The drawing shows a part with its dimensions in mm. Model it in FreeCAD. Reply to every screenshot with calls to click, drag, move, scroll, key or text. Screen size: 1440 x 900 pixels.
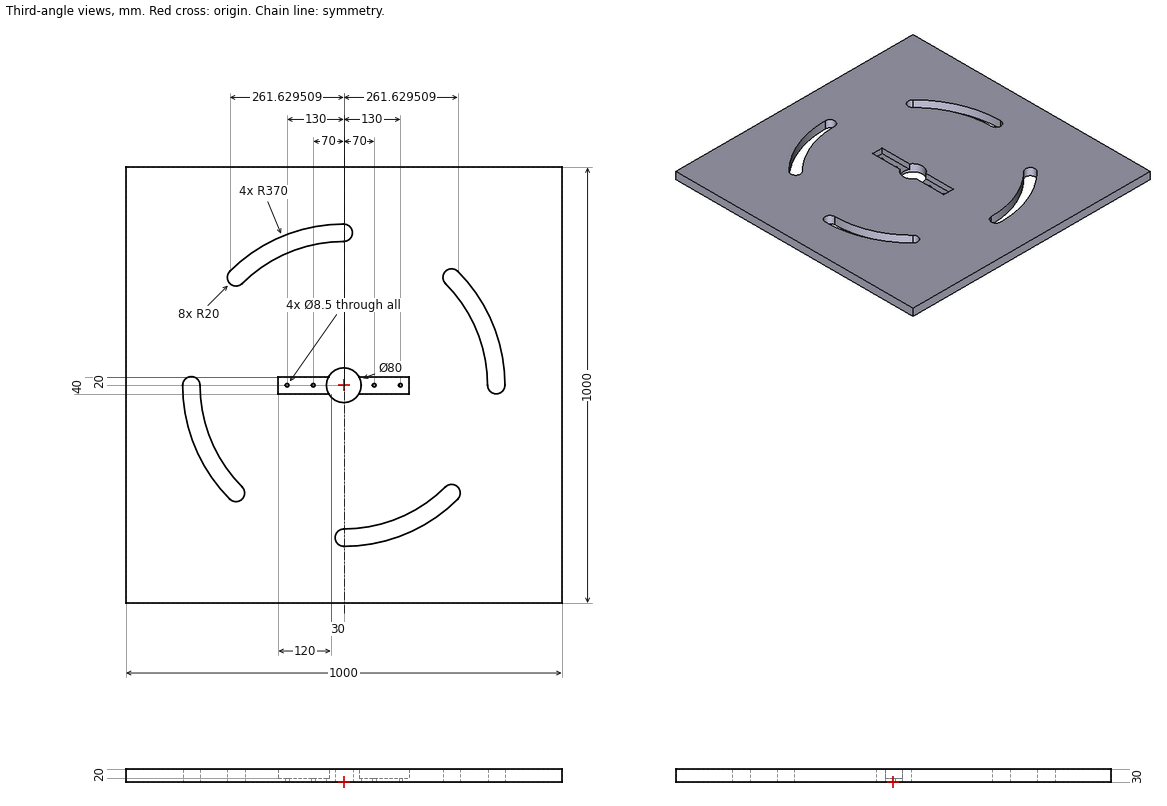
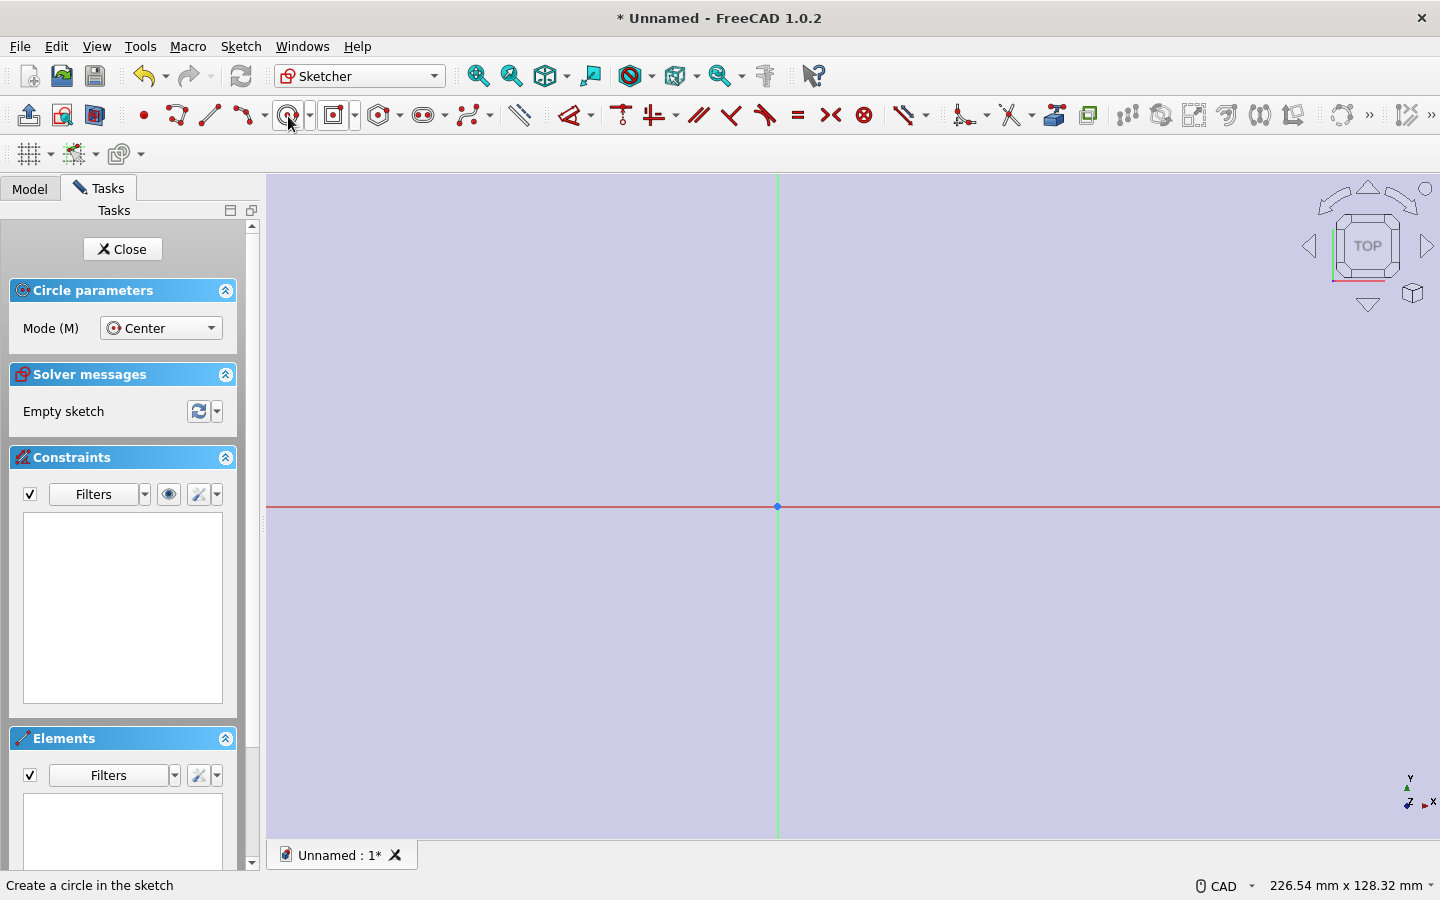
click(778, 506)
click(924, 360)
key(Escape)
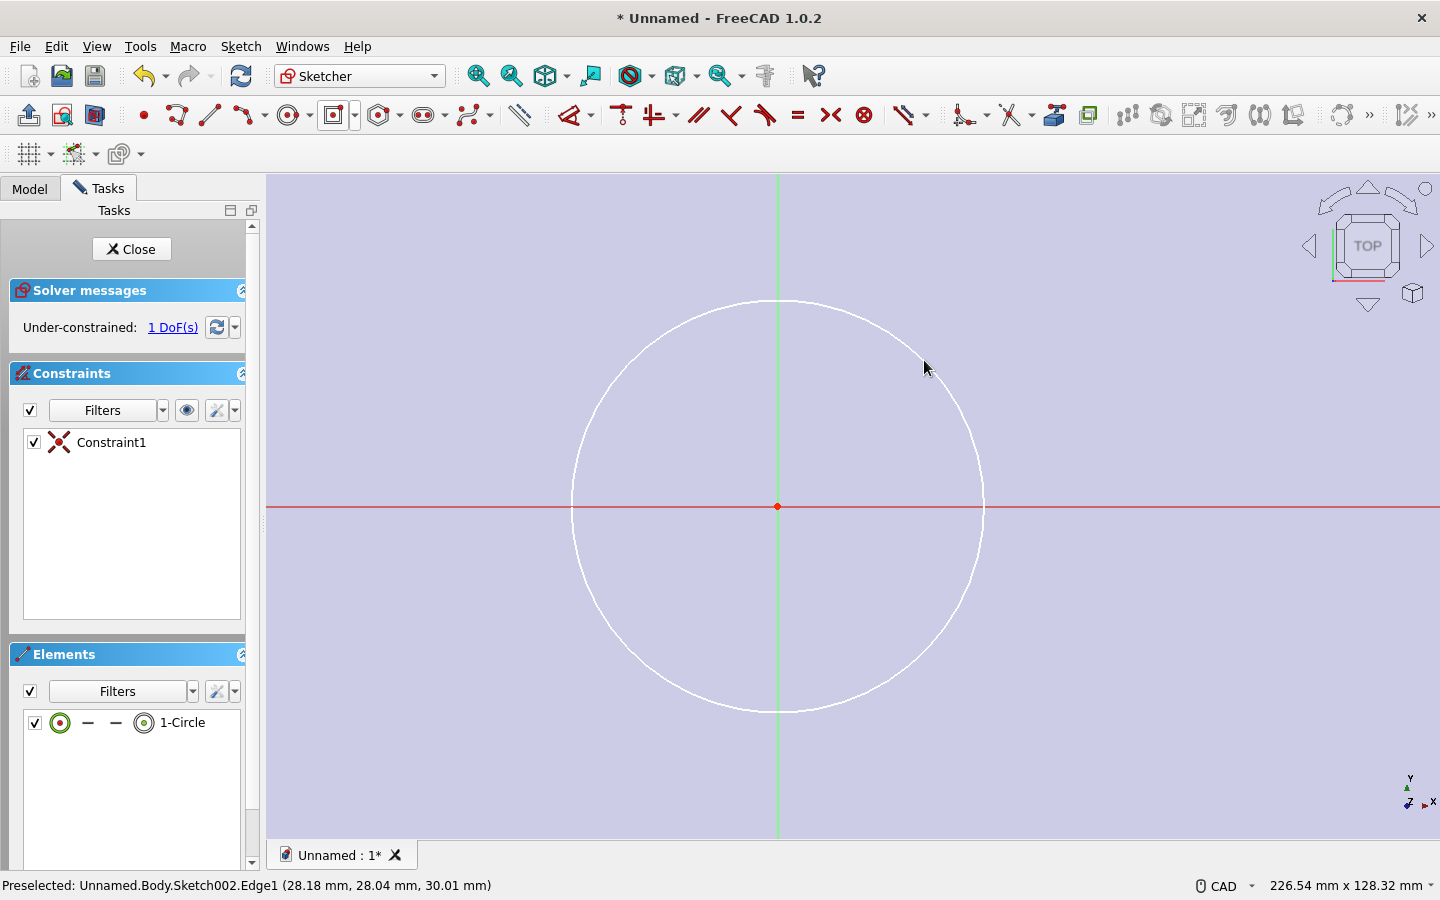
click(568, 116)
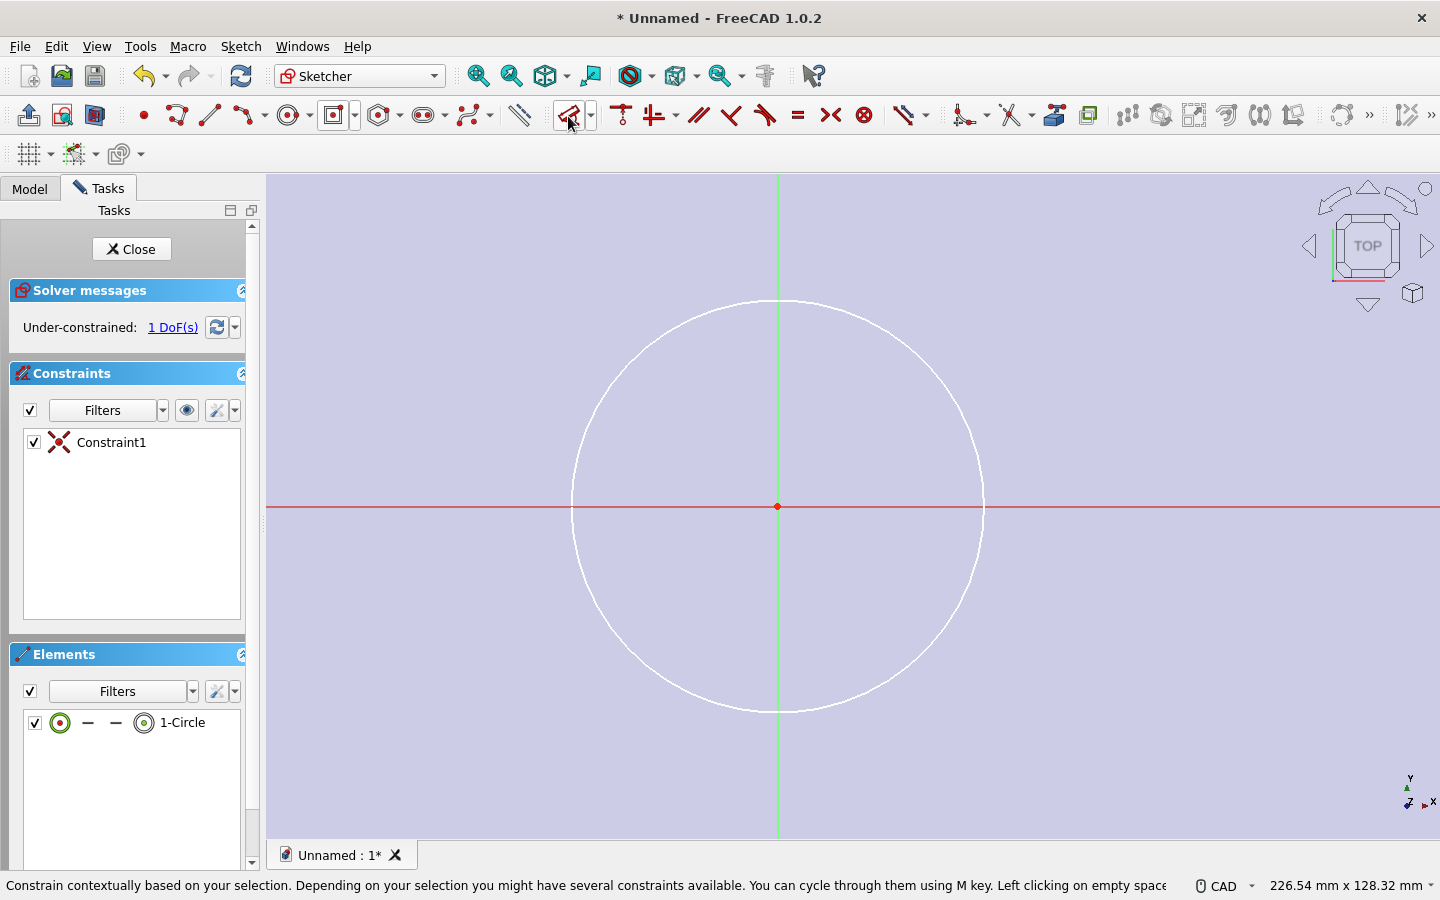
click(923, 360)
click(946, 337)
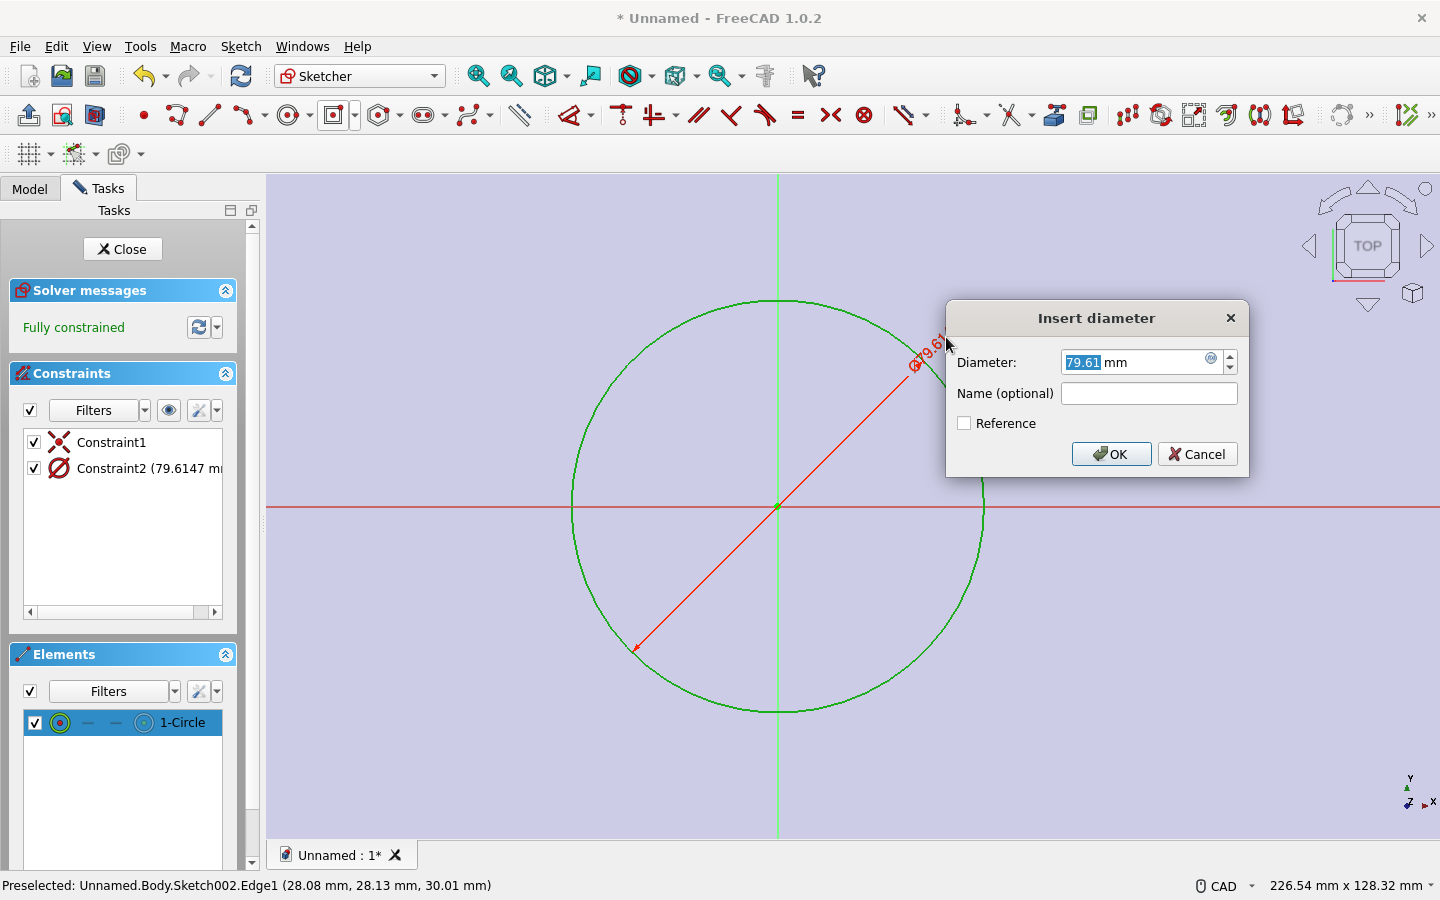
text(80)
key(Return)
key(Escape)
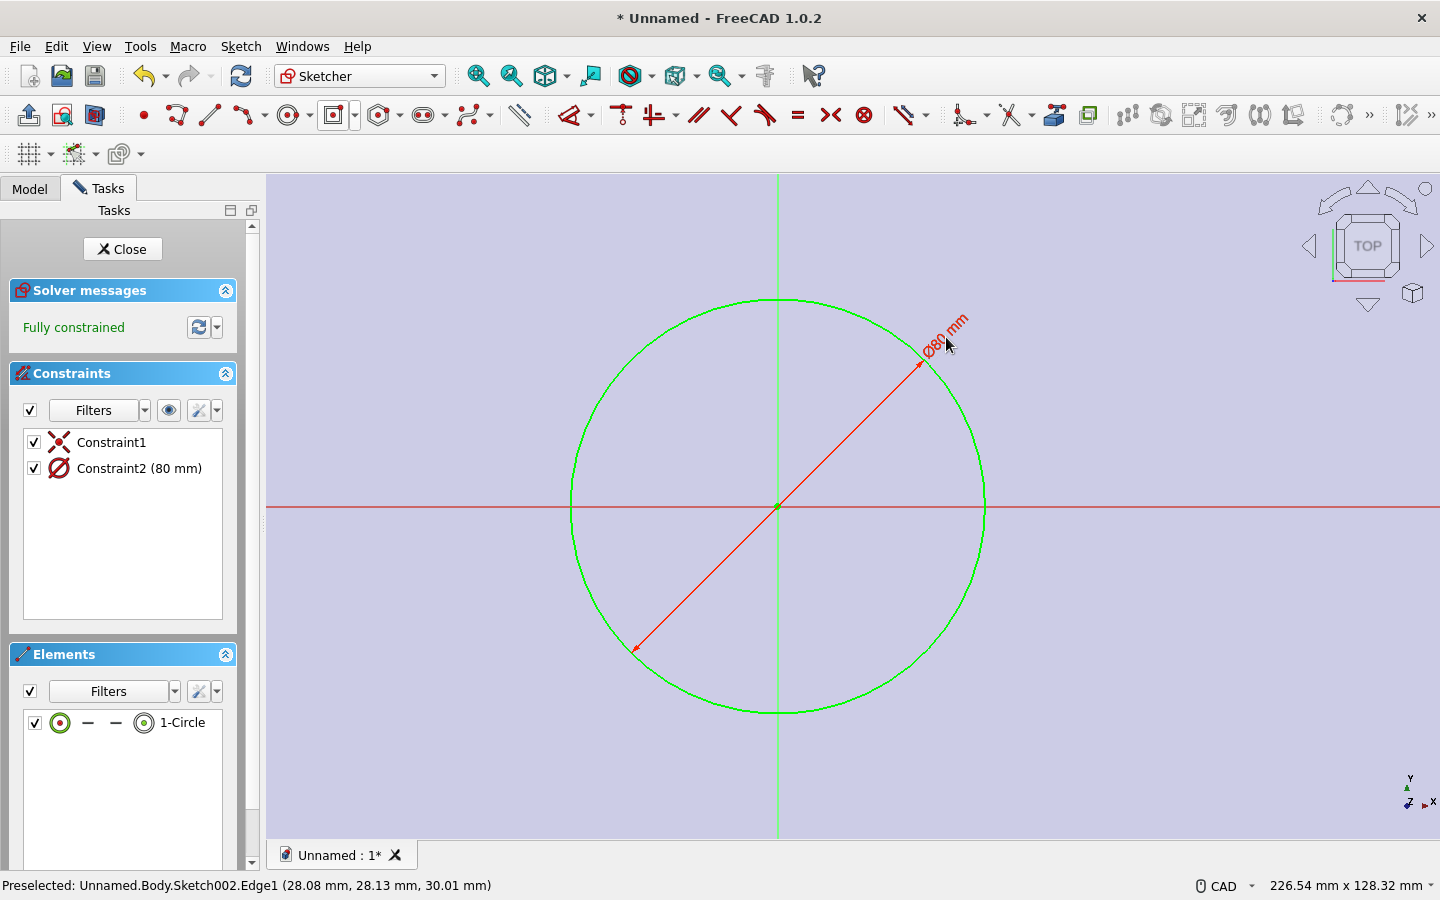
click(123, 249)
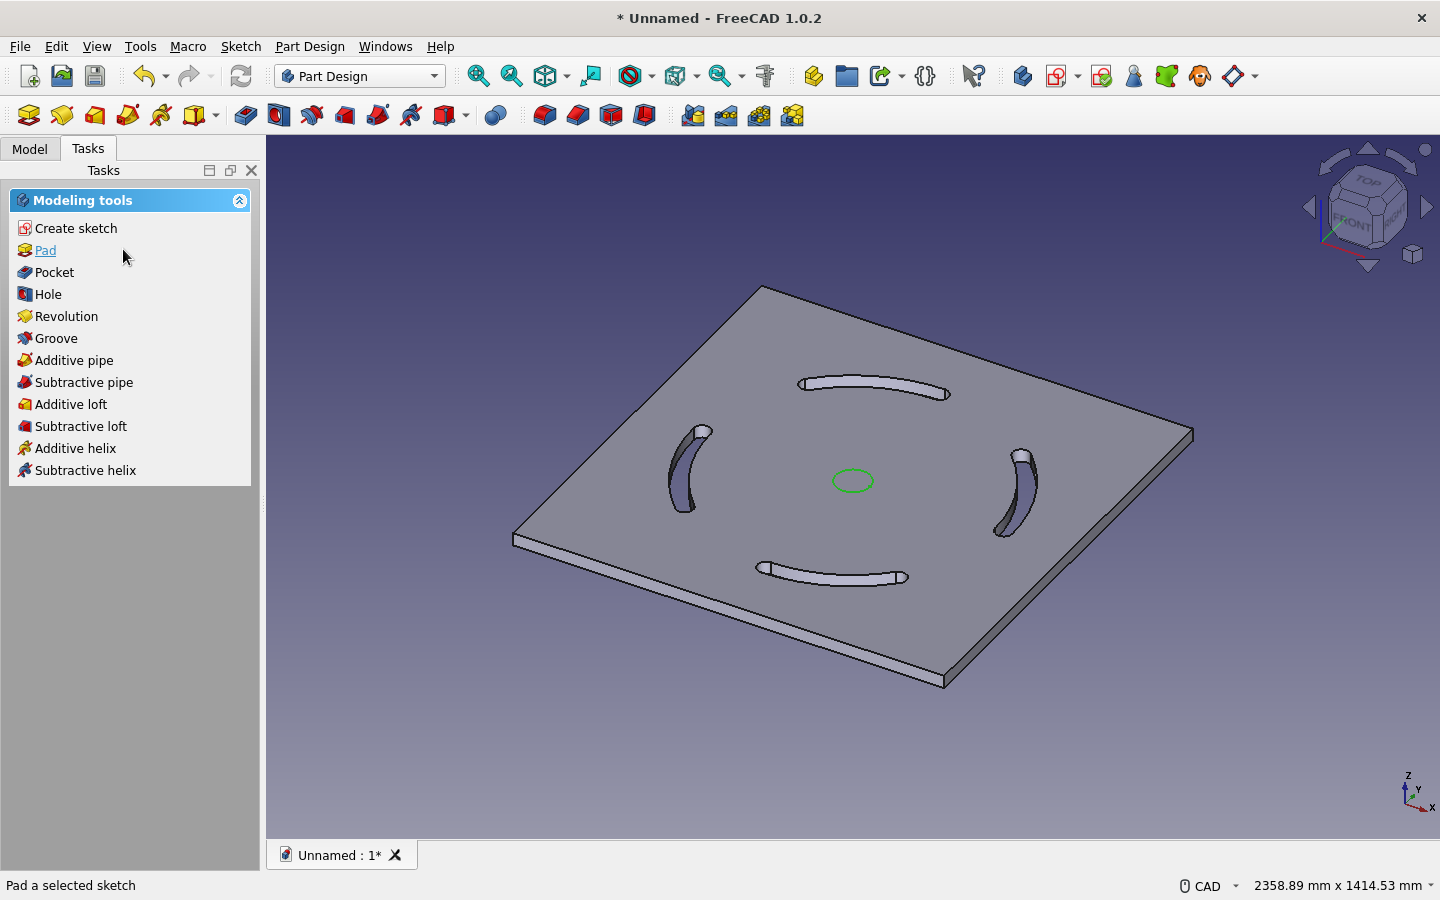
click(246, 116)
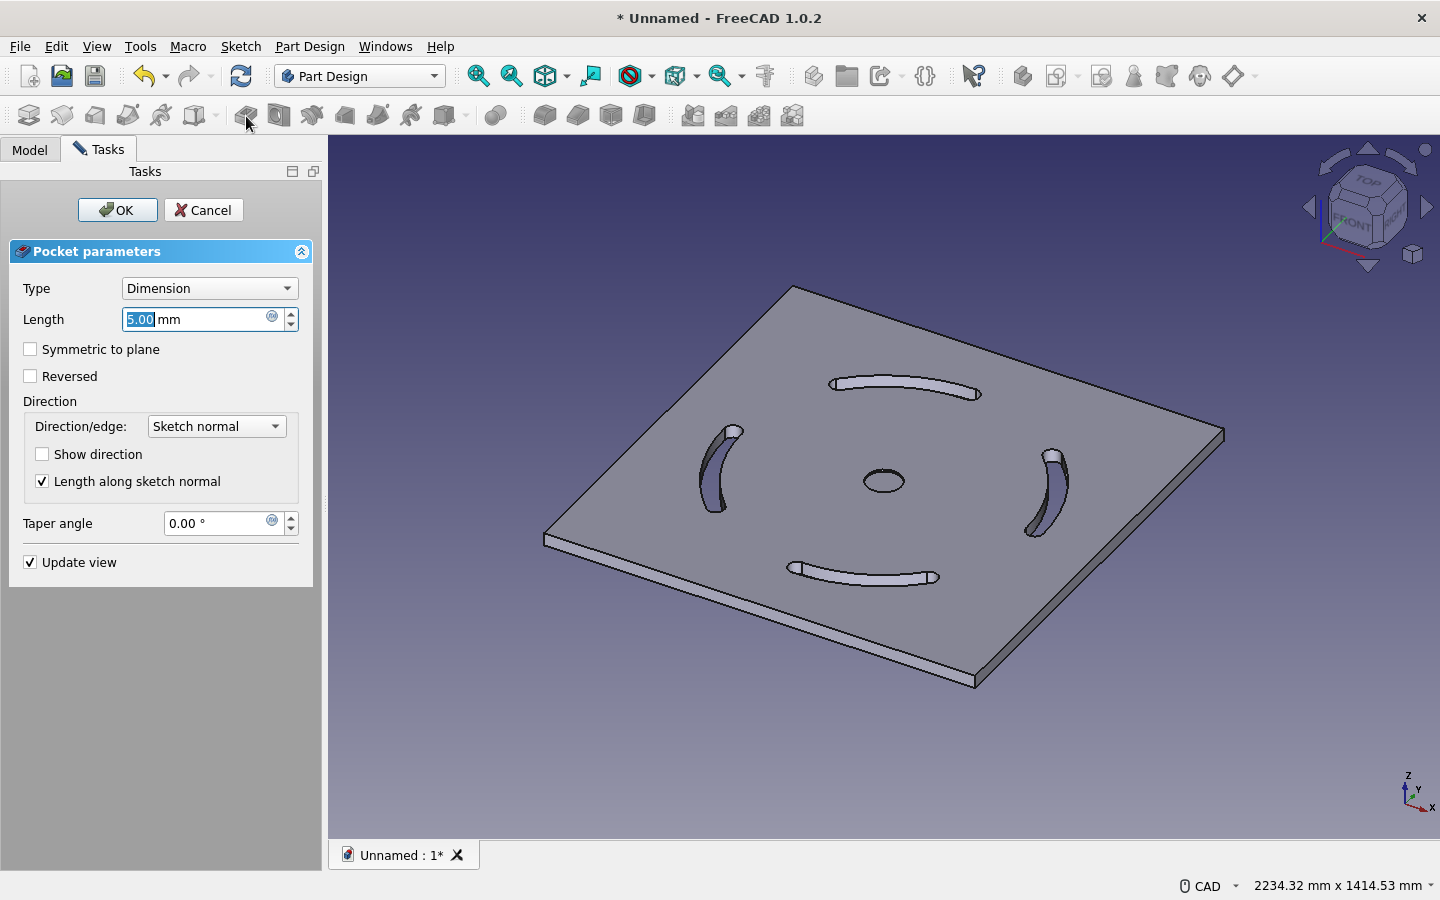
click(210, 288)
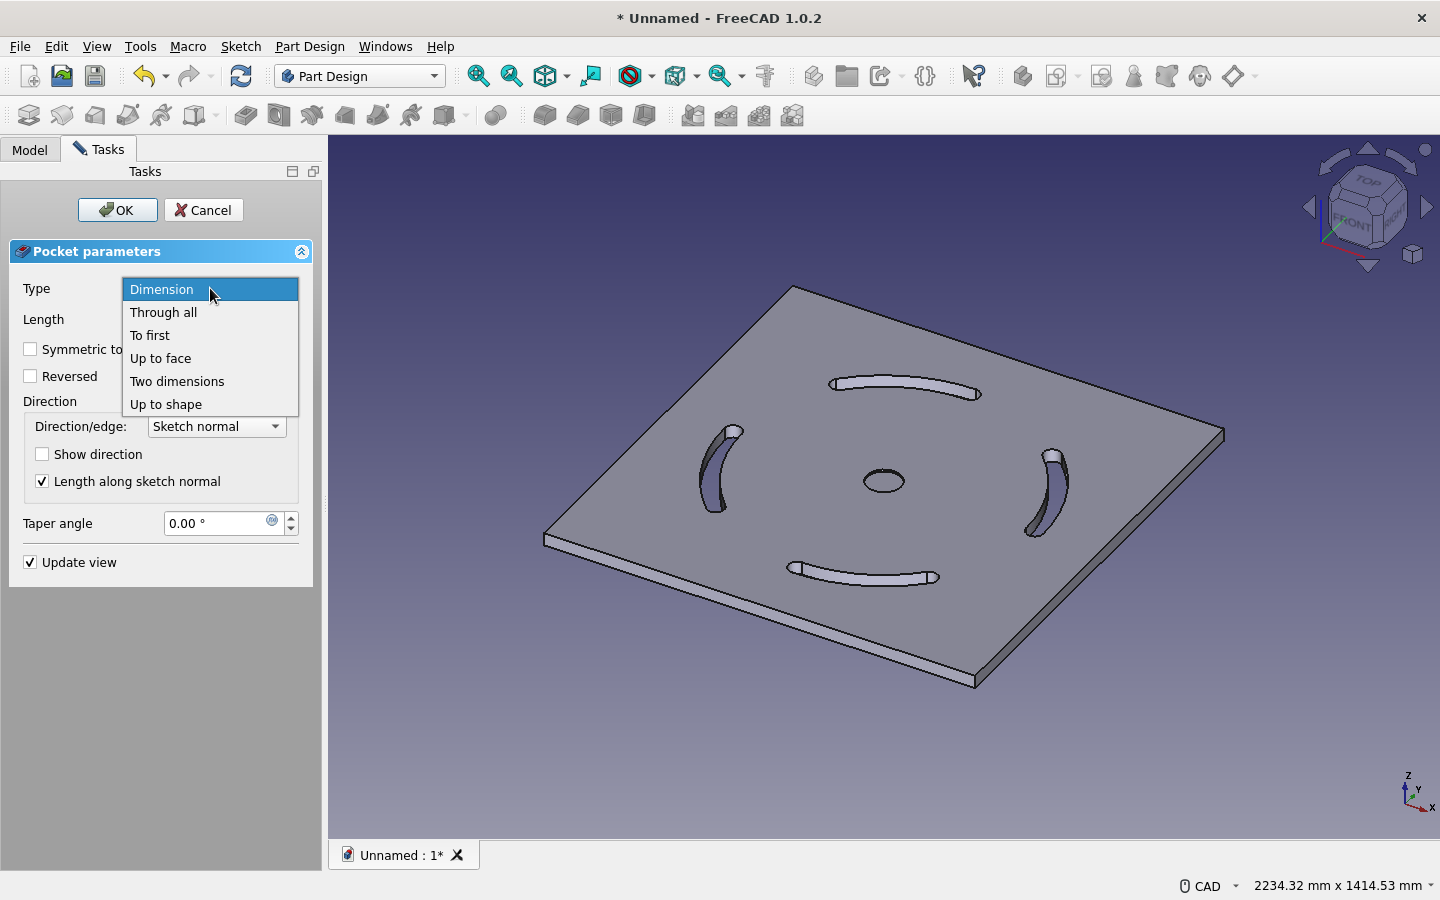
click(208, 312)